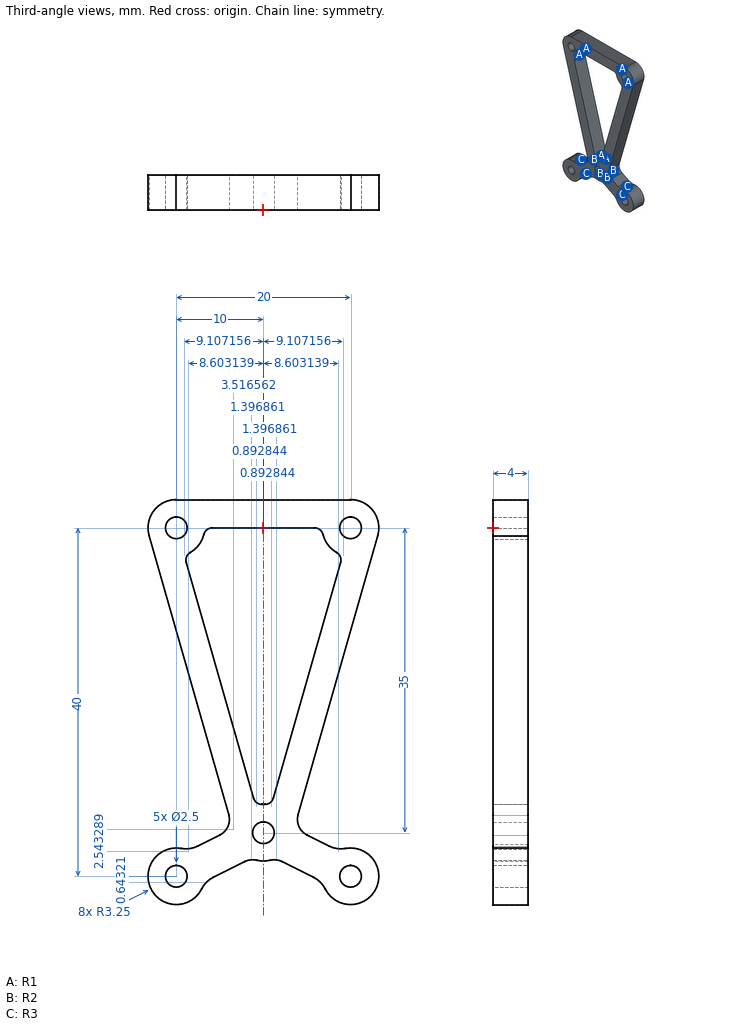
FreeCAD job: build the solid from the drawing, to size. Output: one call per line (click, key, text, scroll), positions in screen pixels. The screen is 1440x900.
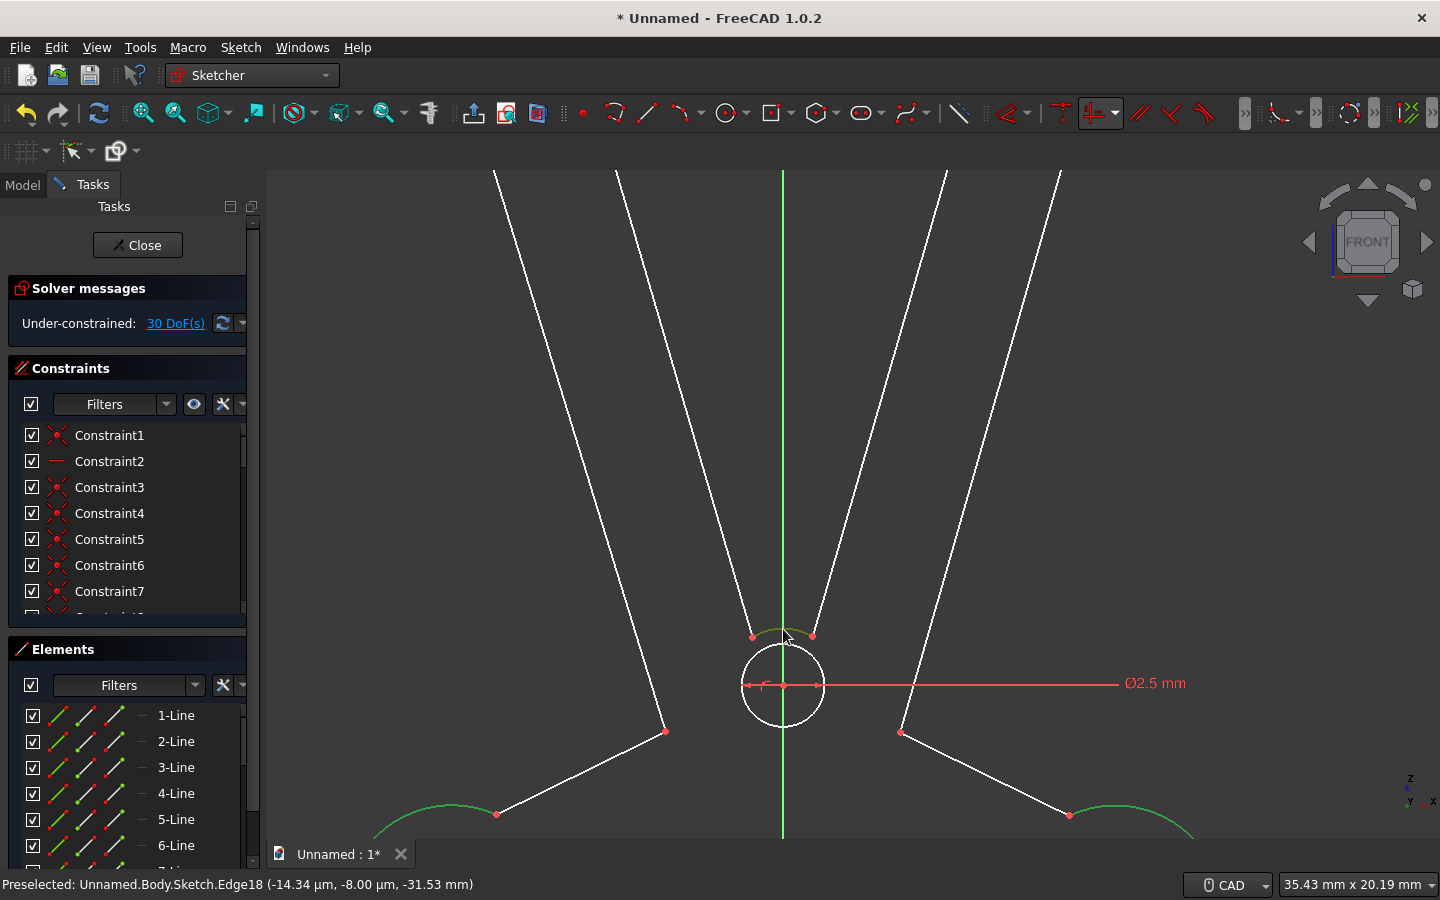
key(e)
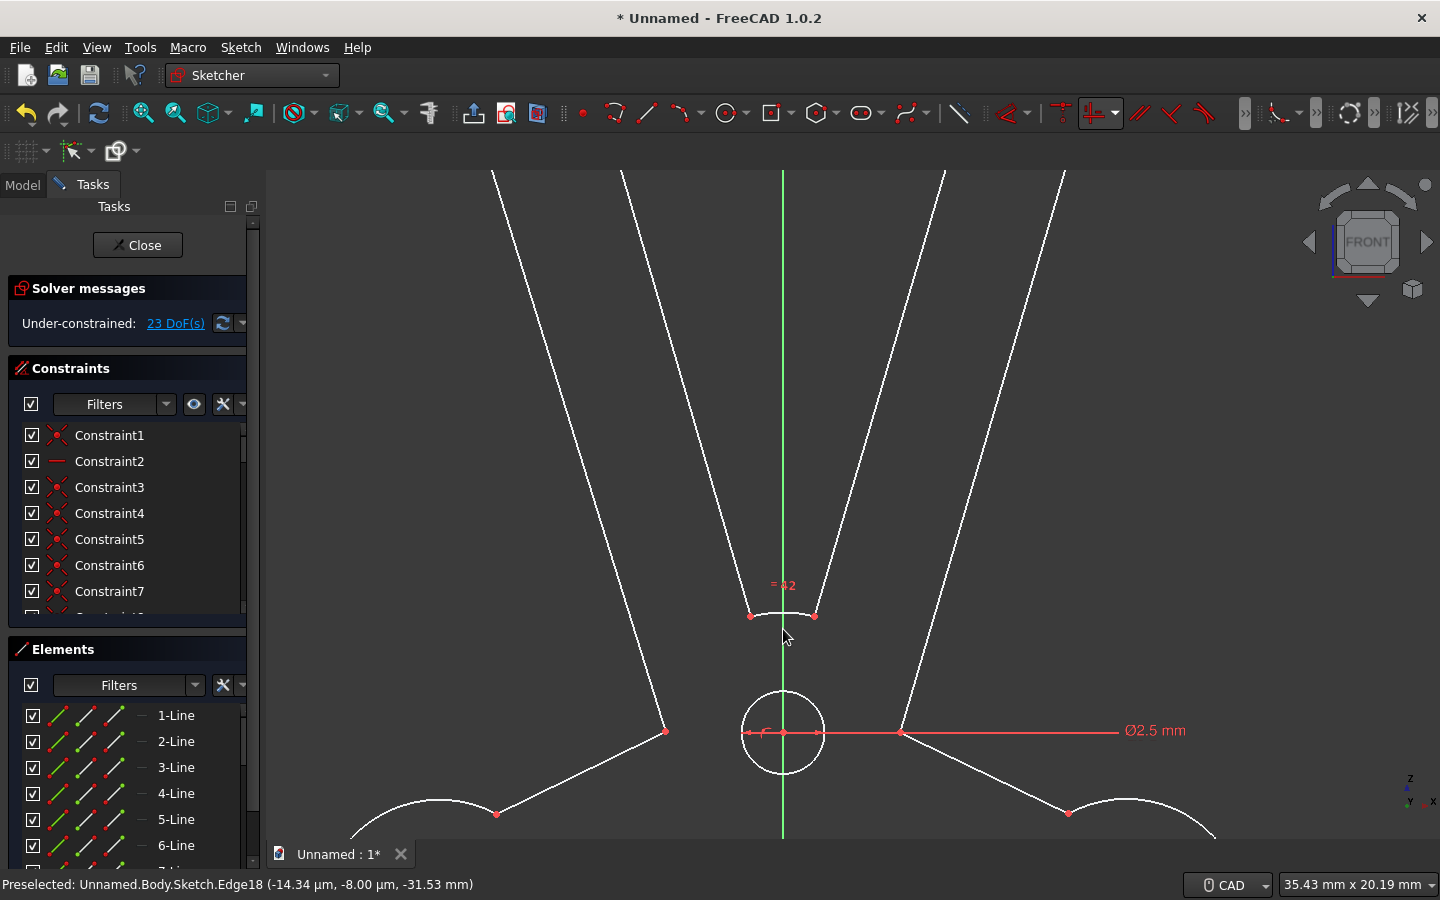
scroll(785, 628, down, 6)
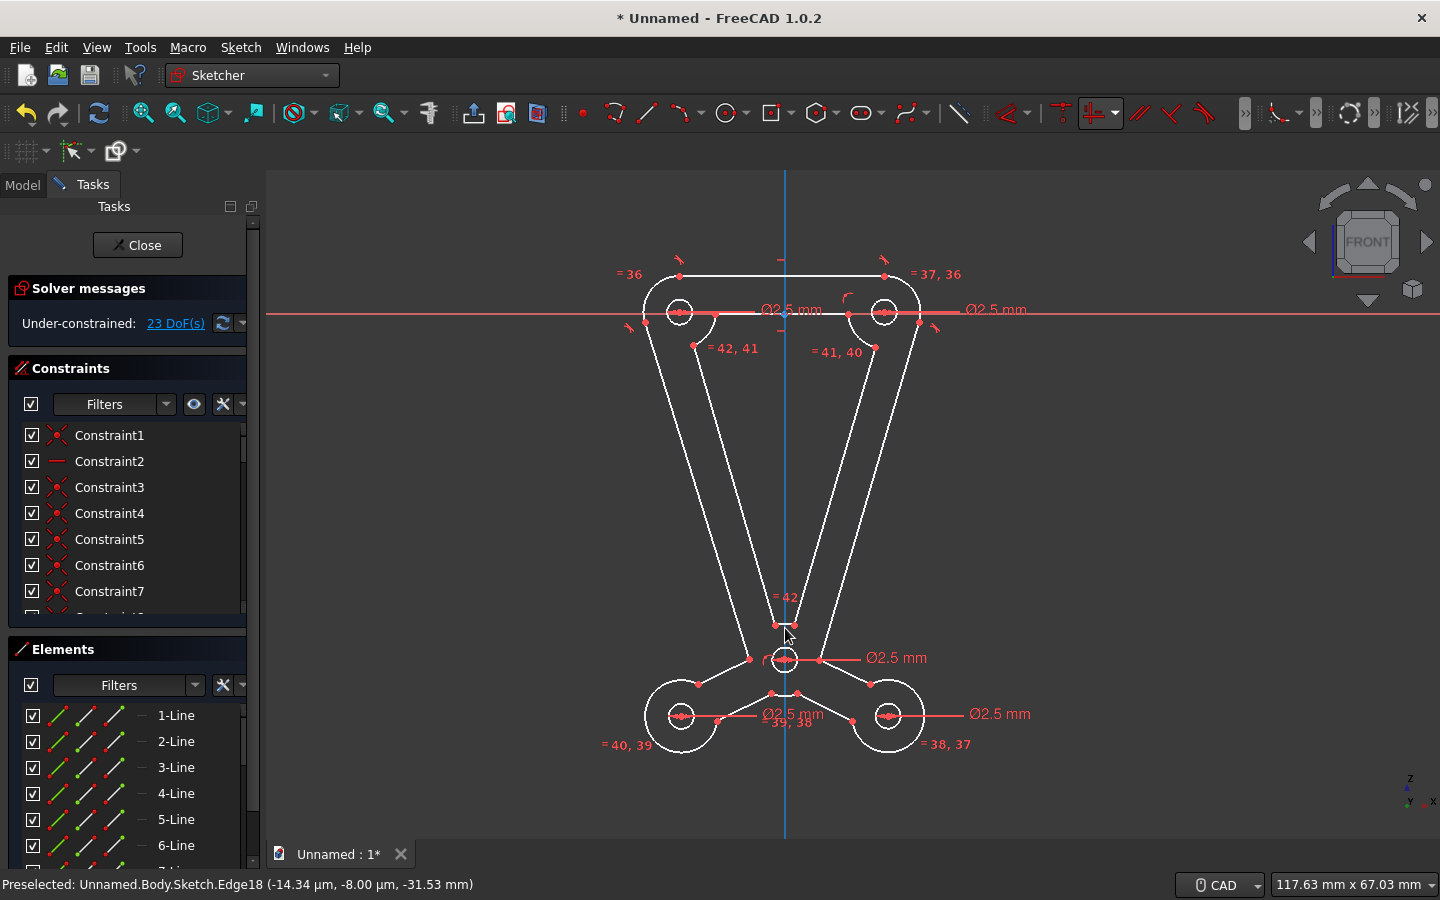
click(680, 312)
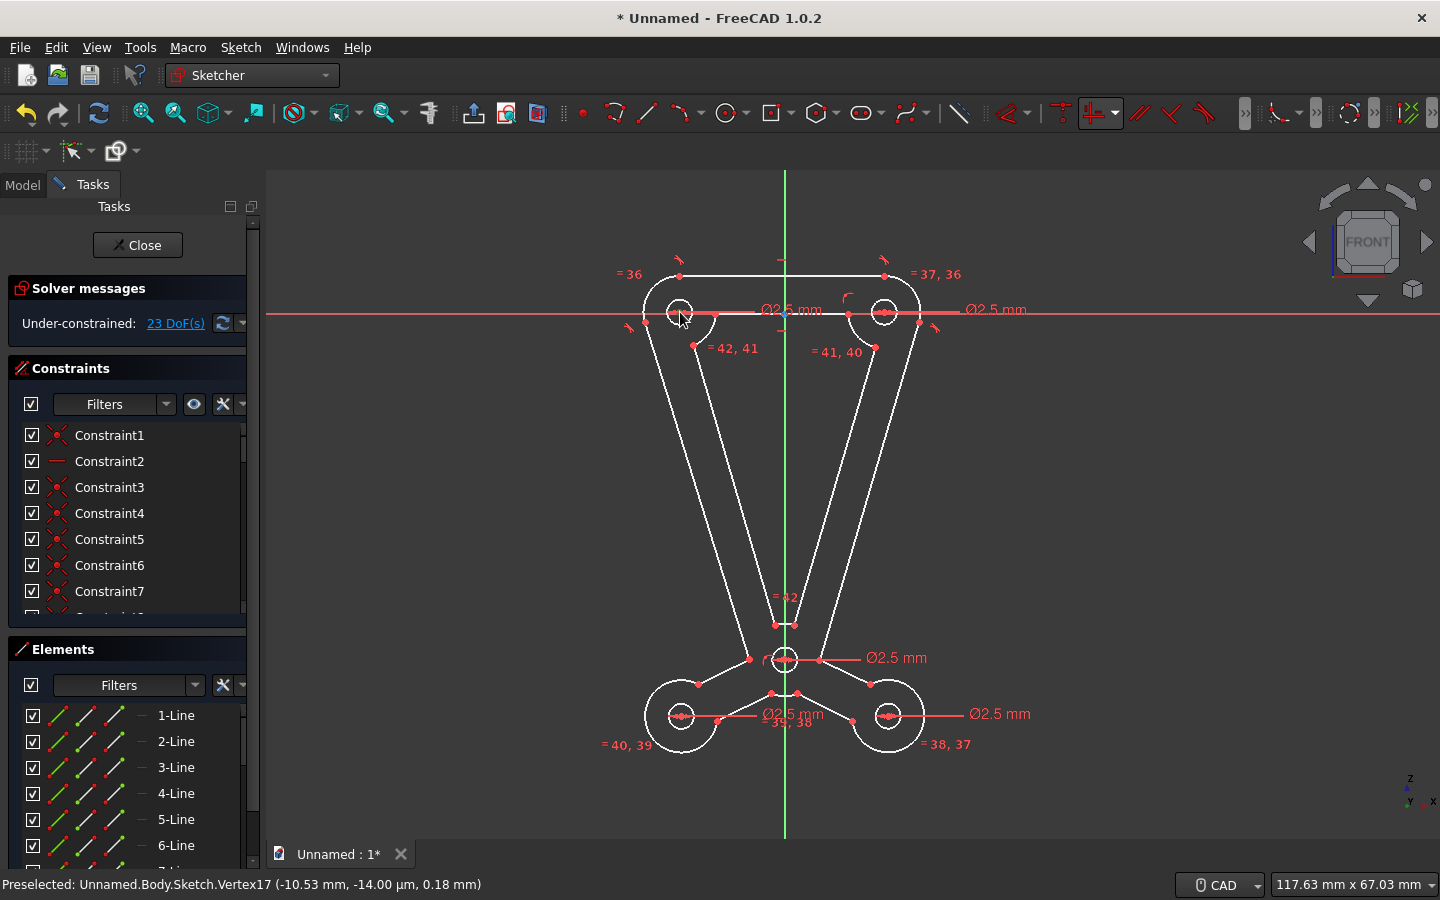
click(364, 314)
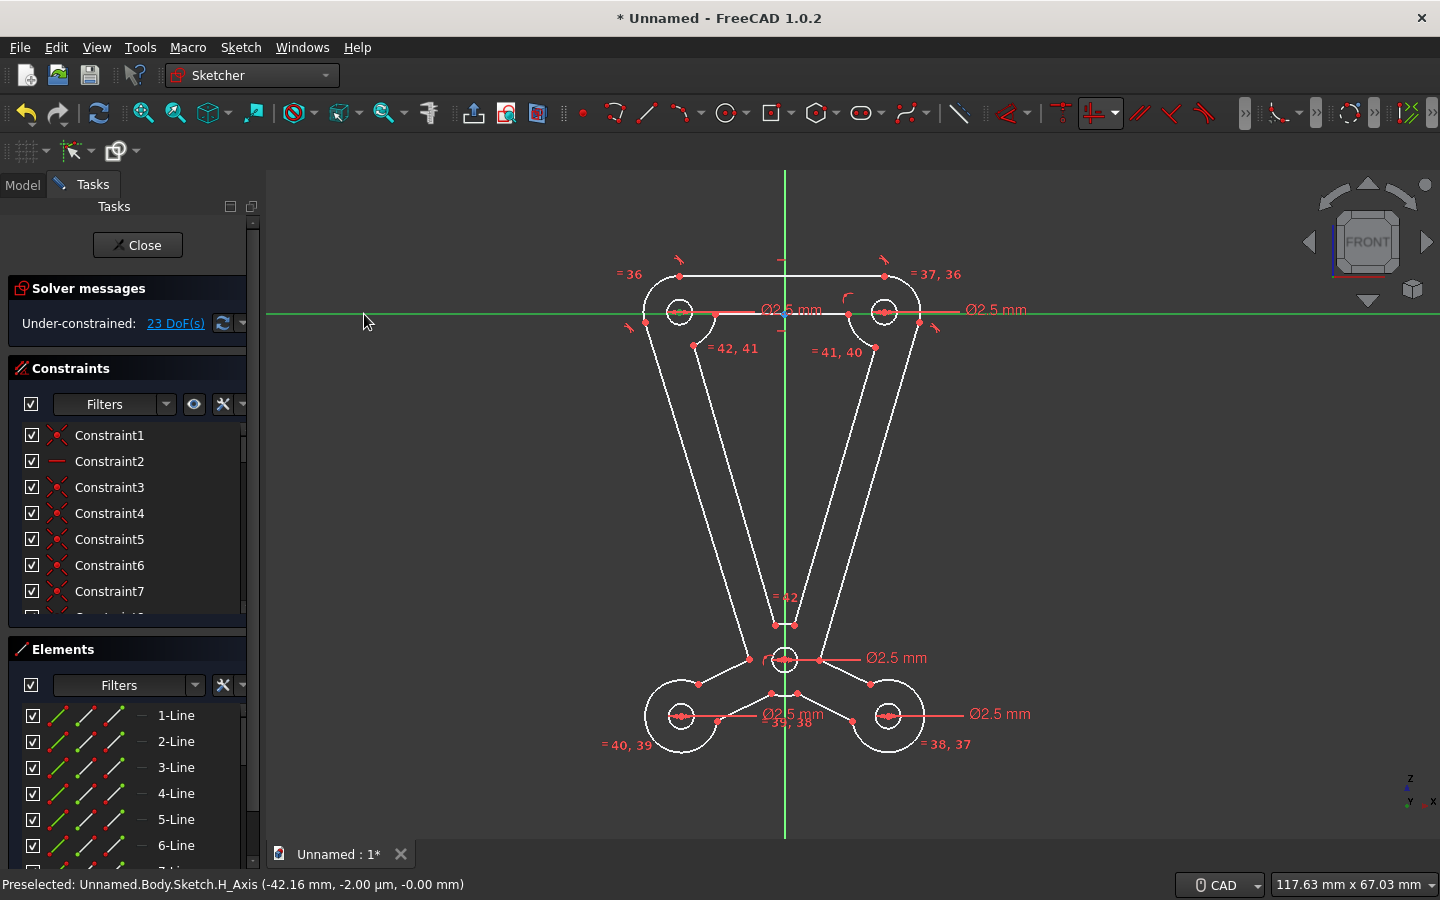
click(1062, 114)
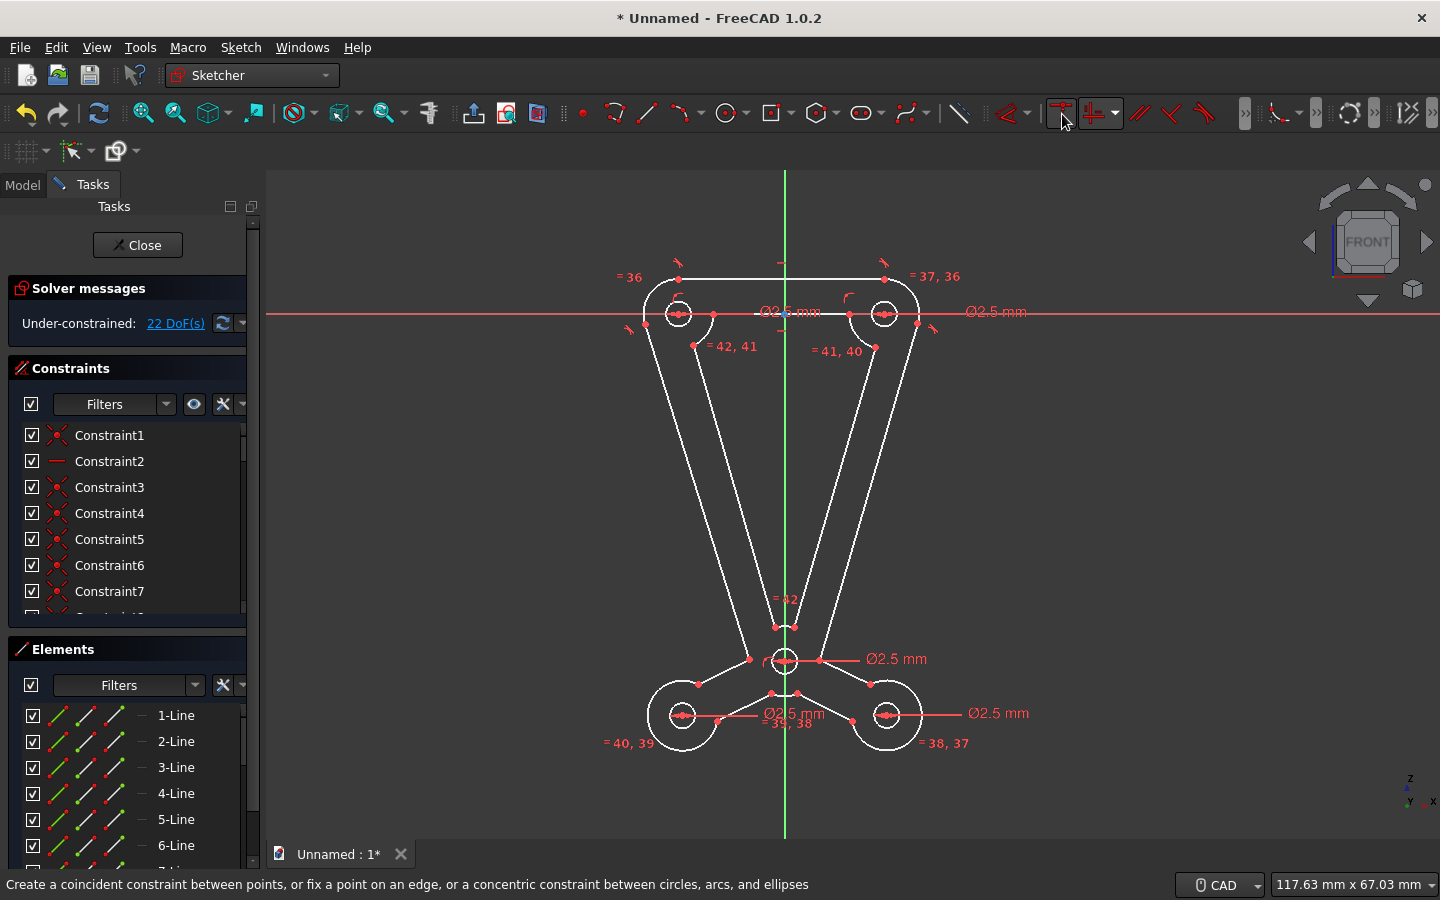
click(887, 715)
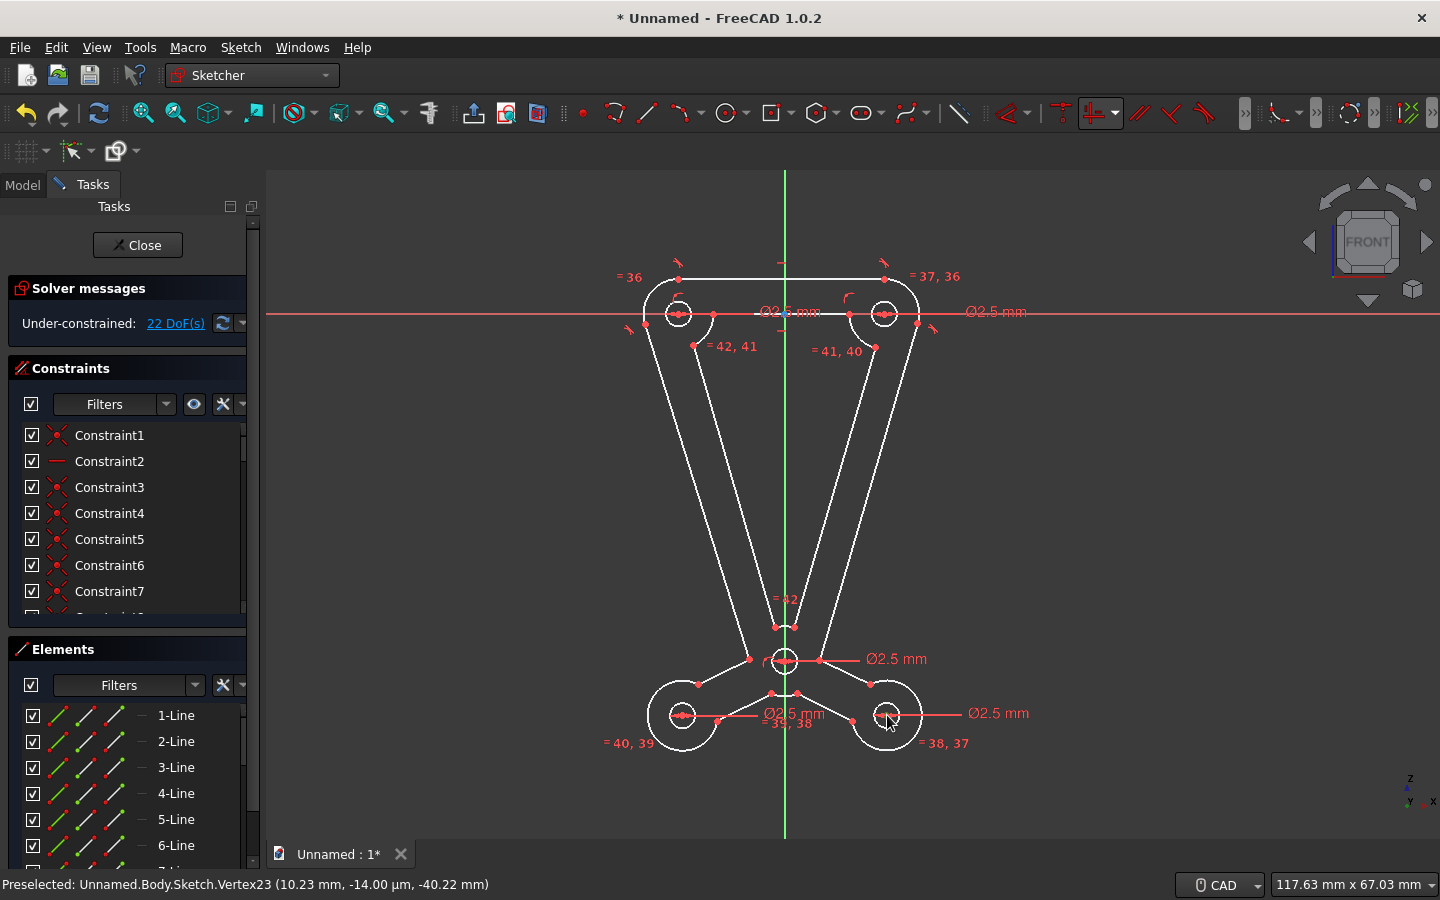
click(683, 716)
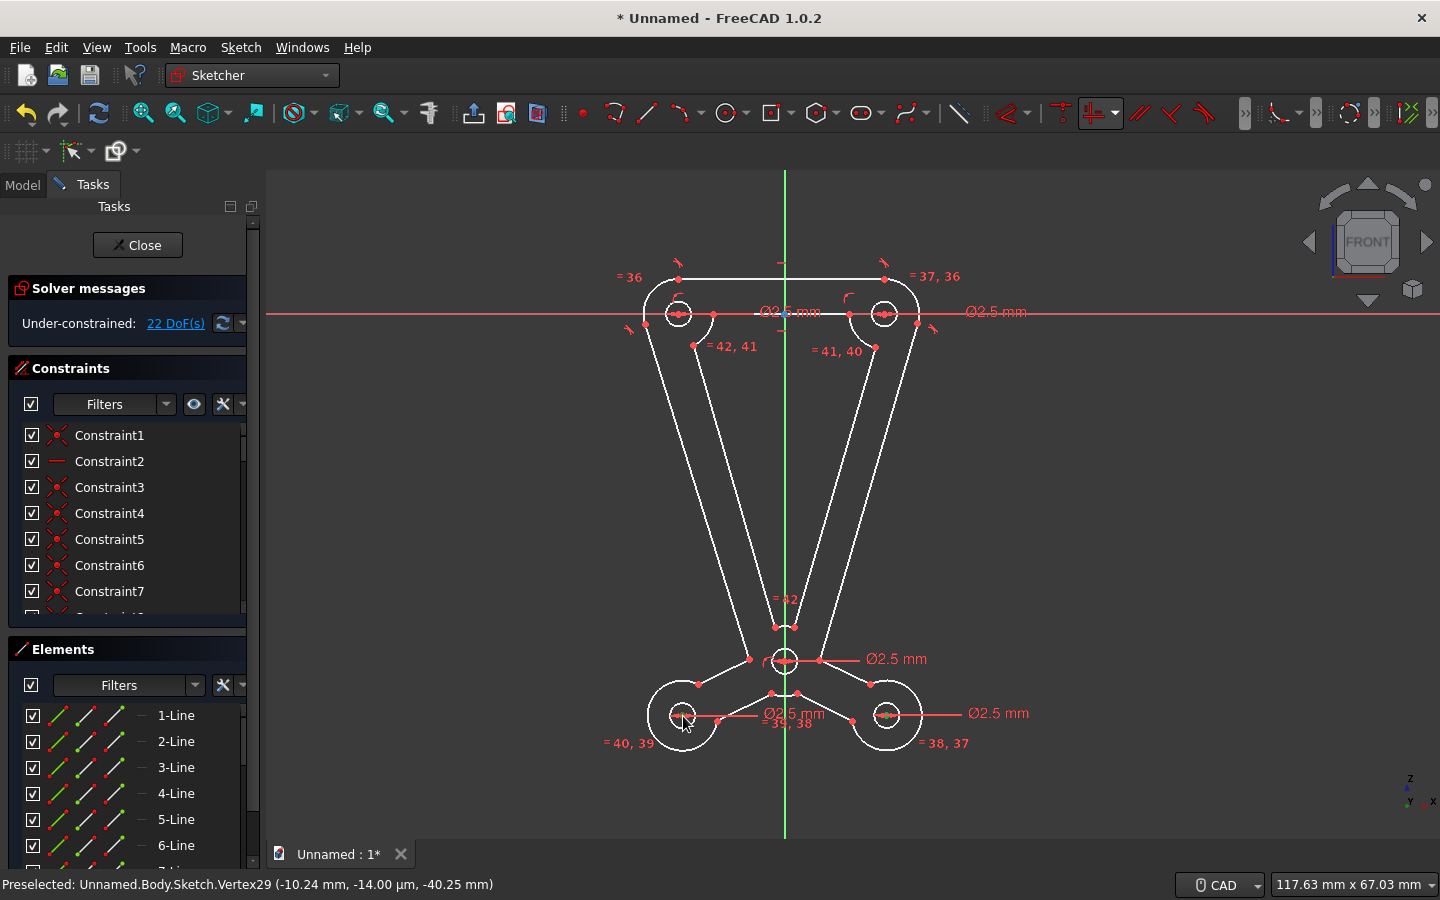
click(785, 767)